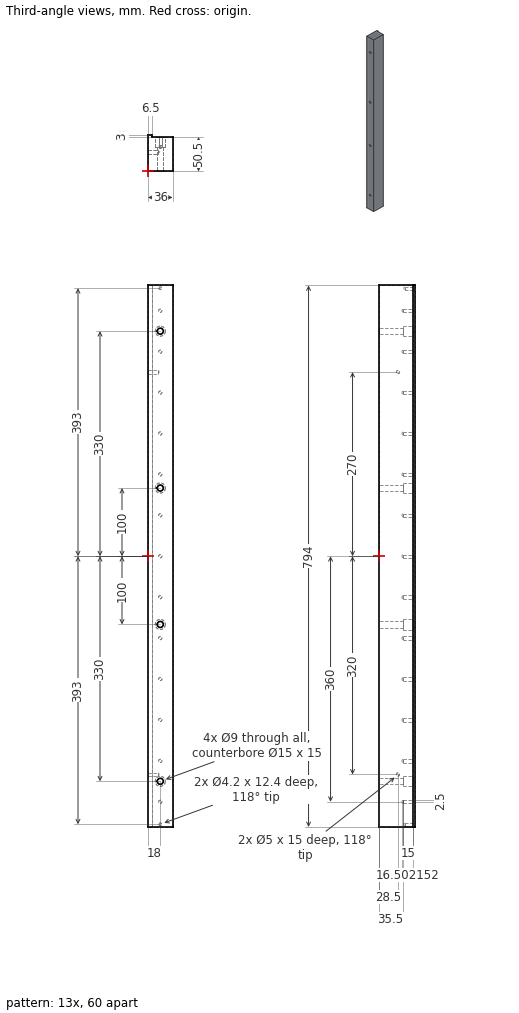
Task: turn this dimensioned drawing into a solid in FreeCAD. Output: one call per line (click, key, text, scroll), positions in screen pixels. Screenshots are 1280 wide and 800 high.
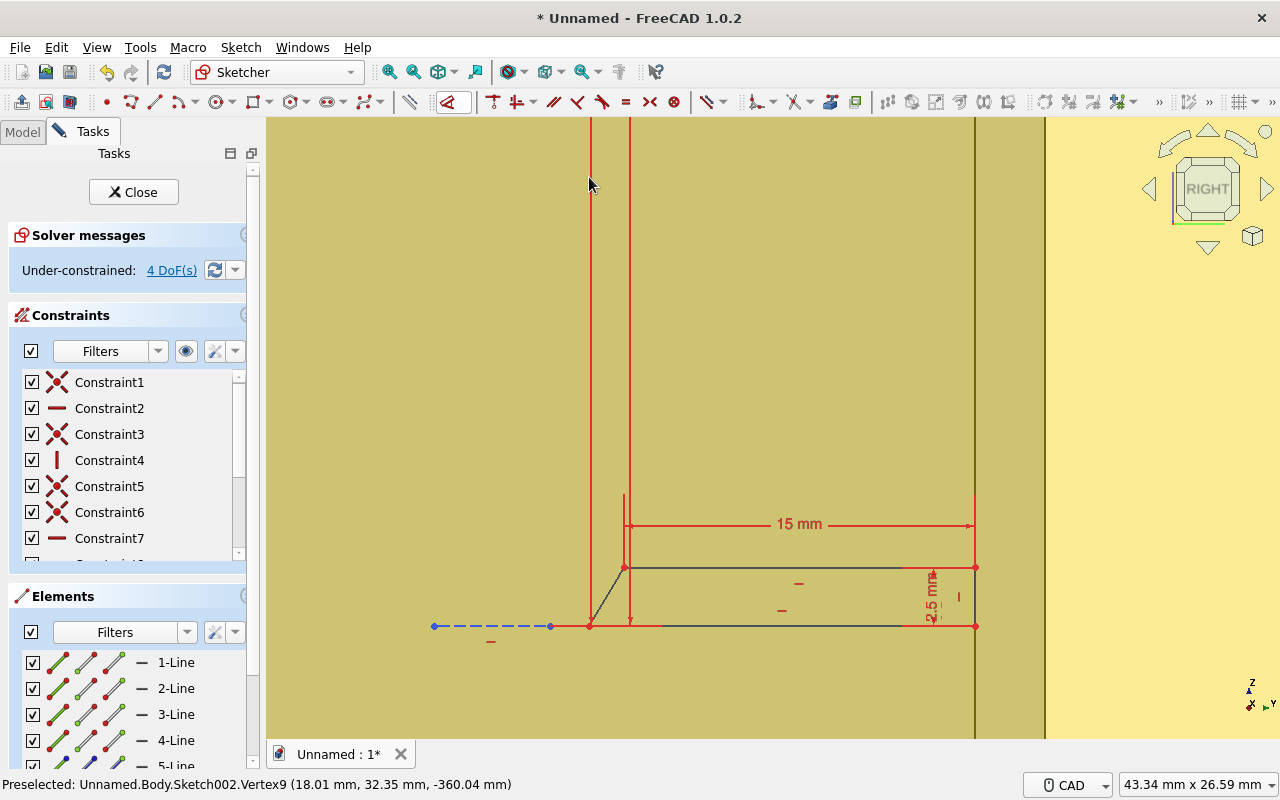
click(624, 568)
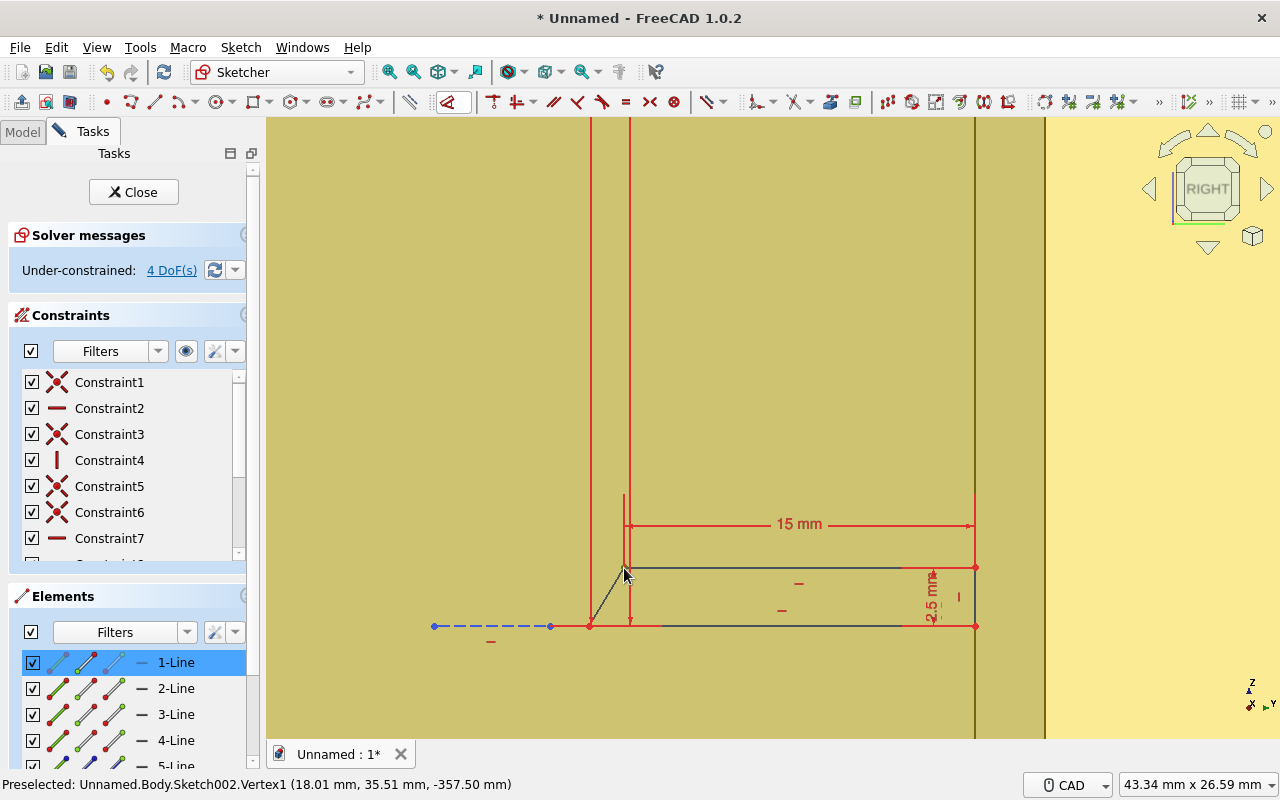
key(l)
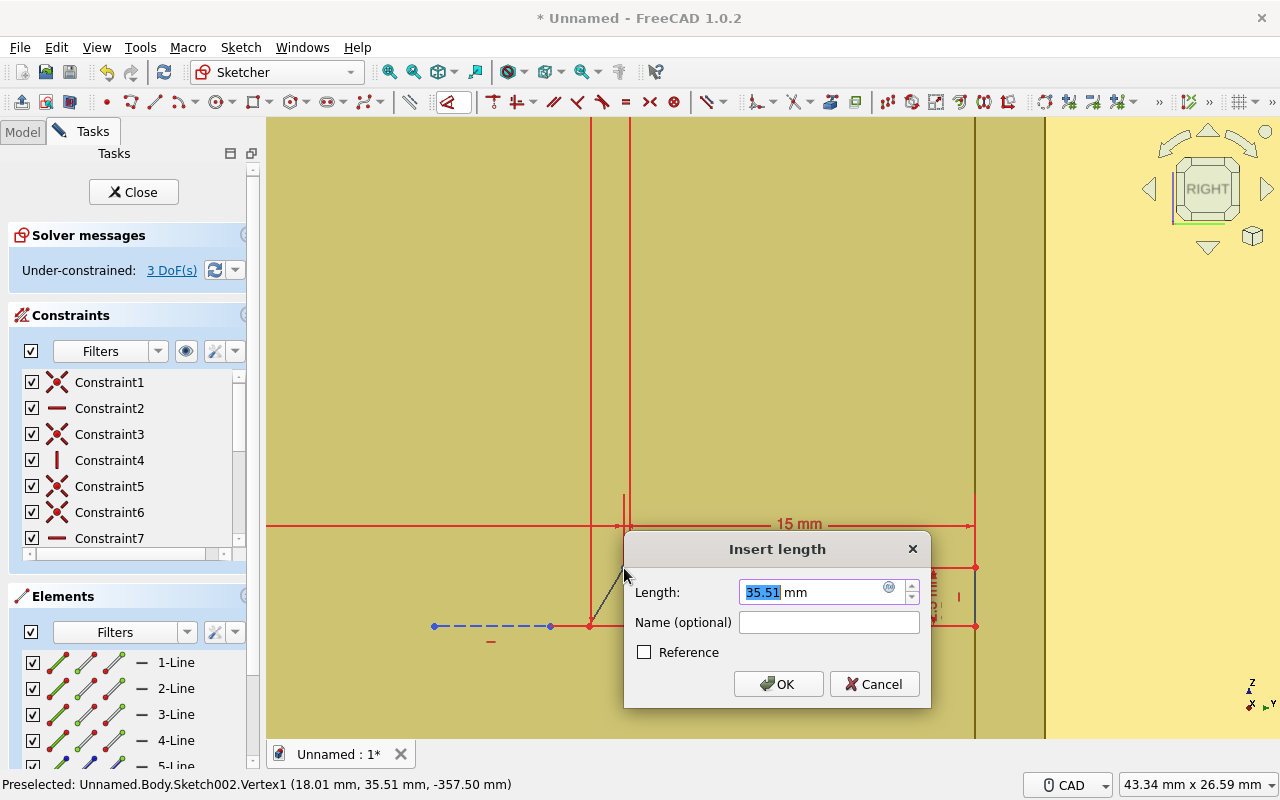
text(35.5)
key(Return)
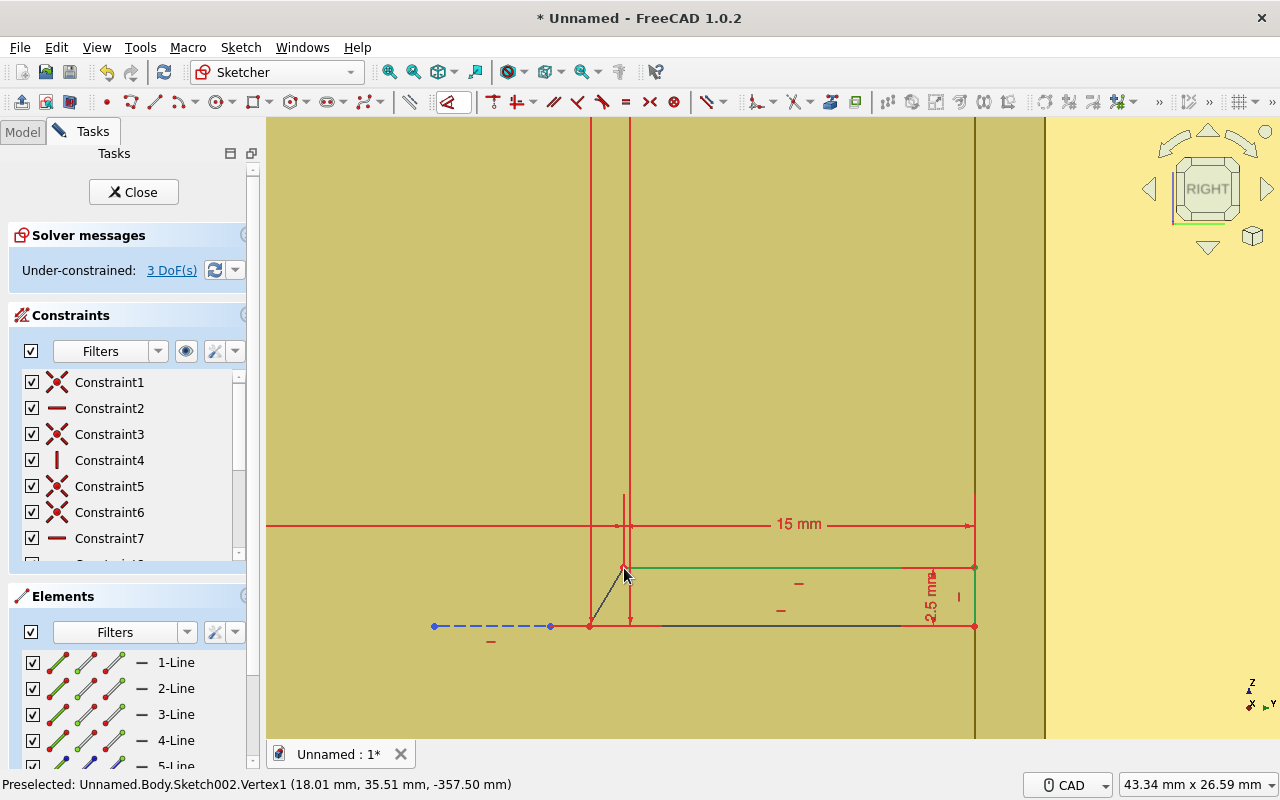
click(705, 626)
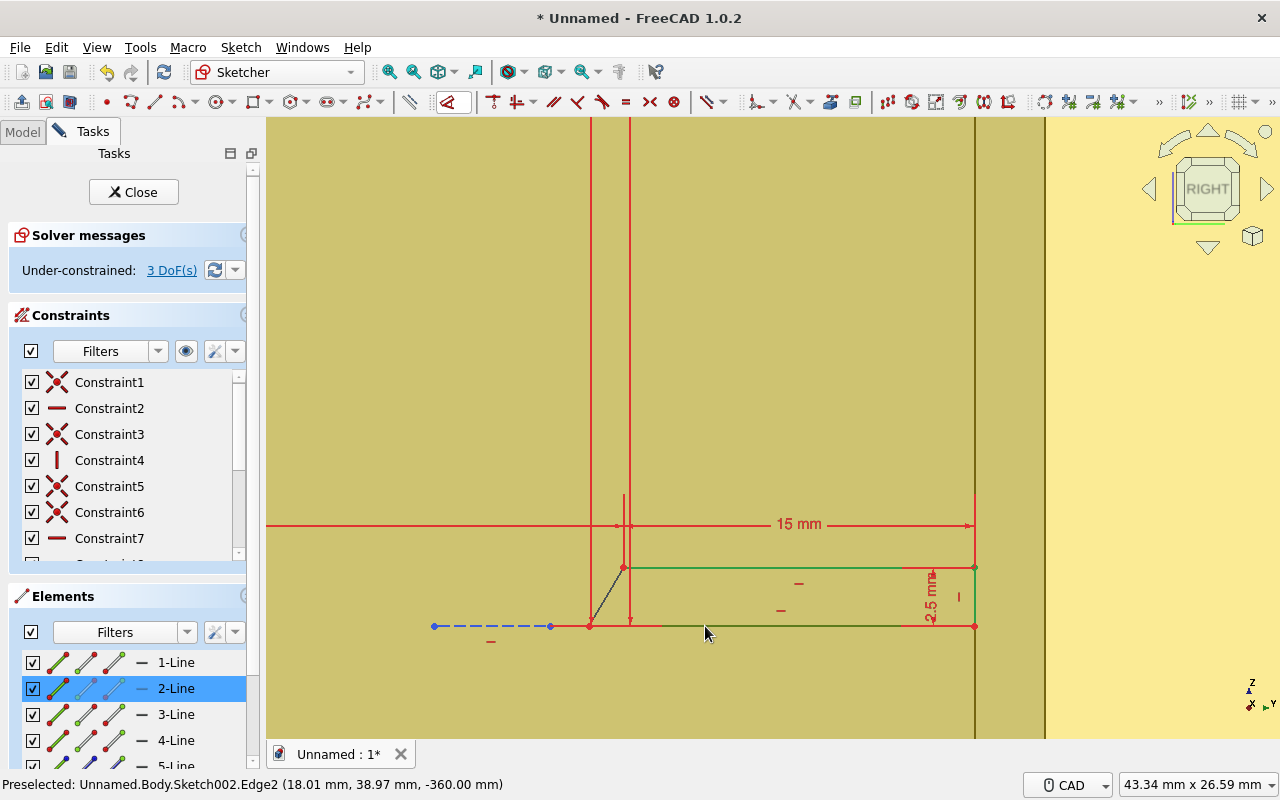
click(466, 102)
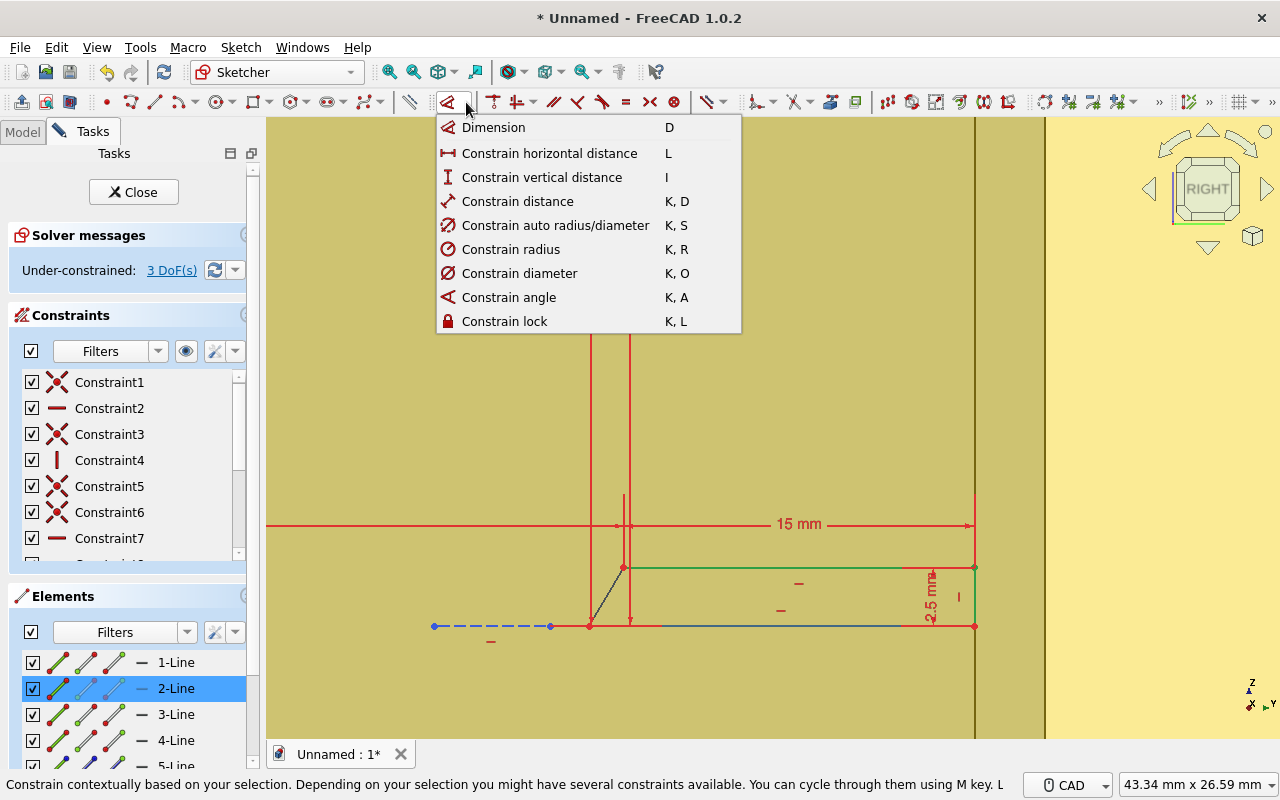
click(589, 153)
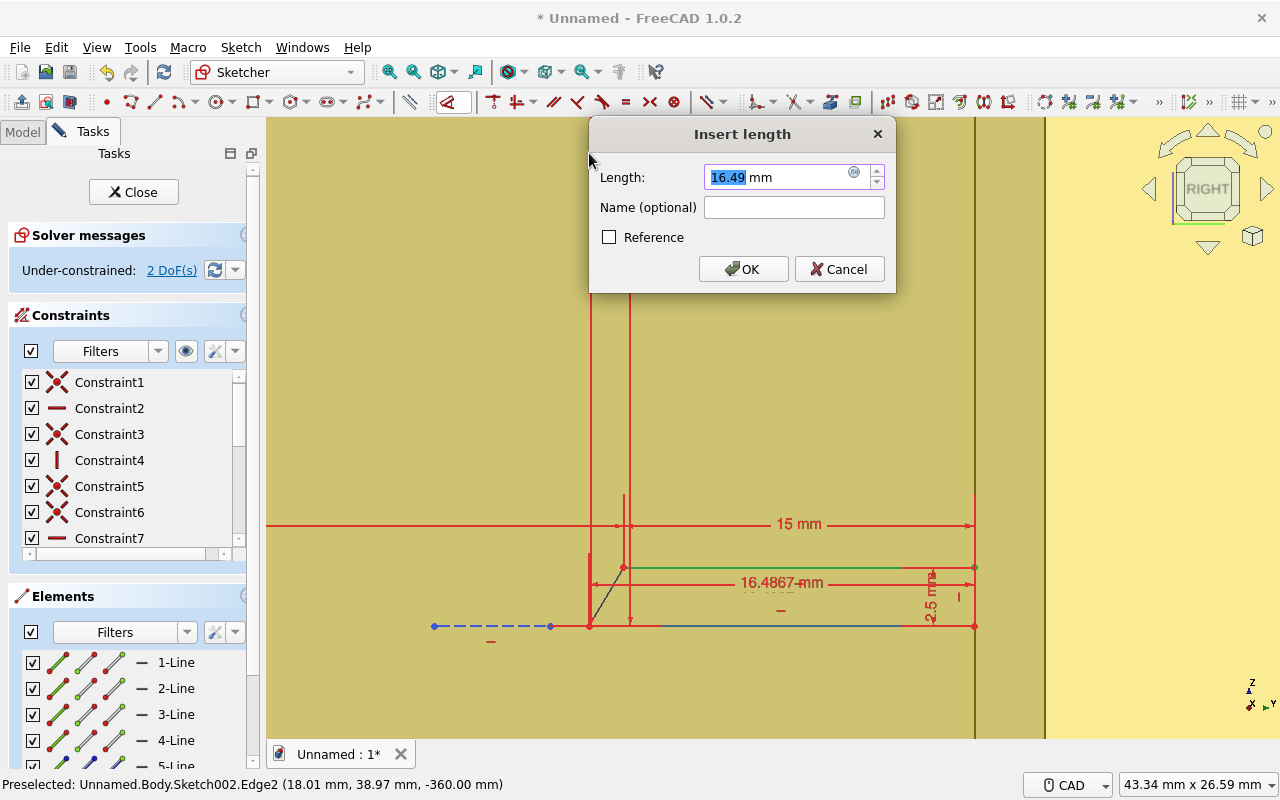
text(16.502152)
key(Return)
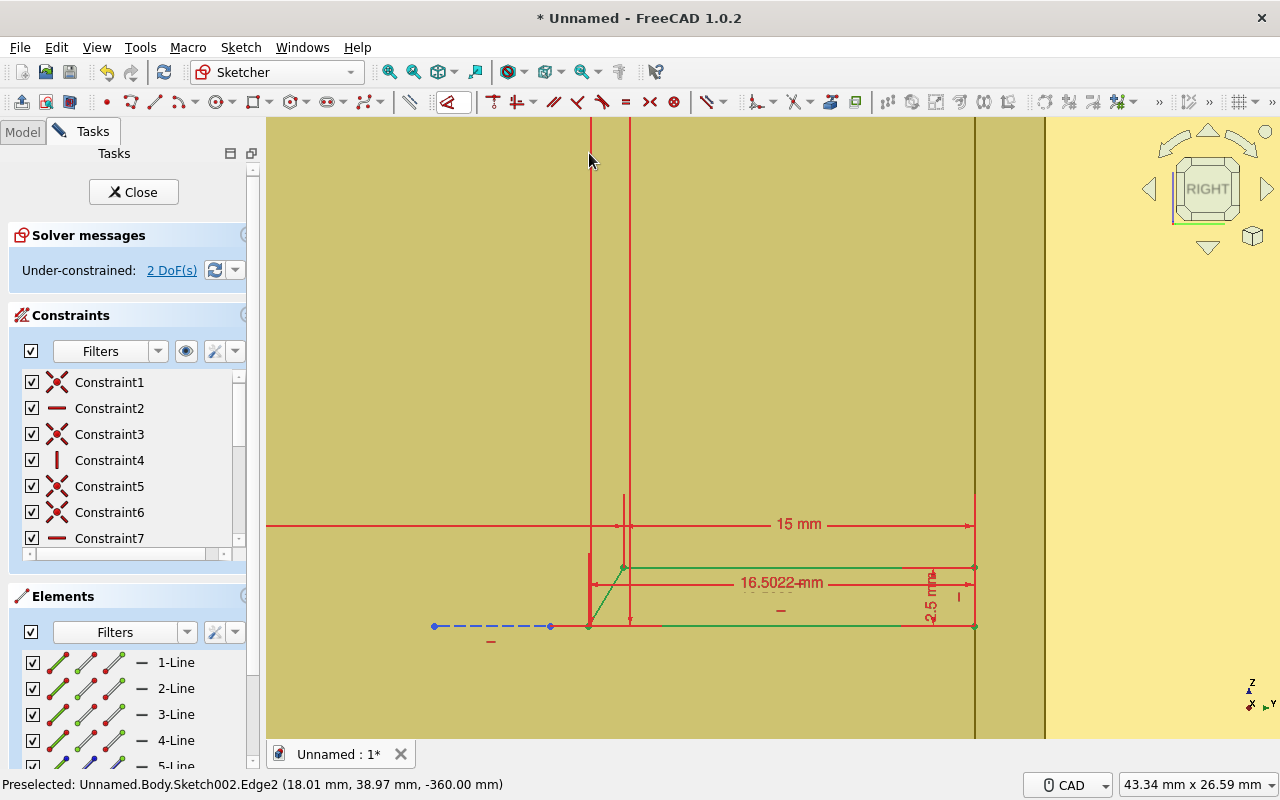
click(134, 192)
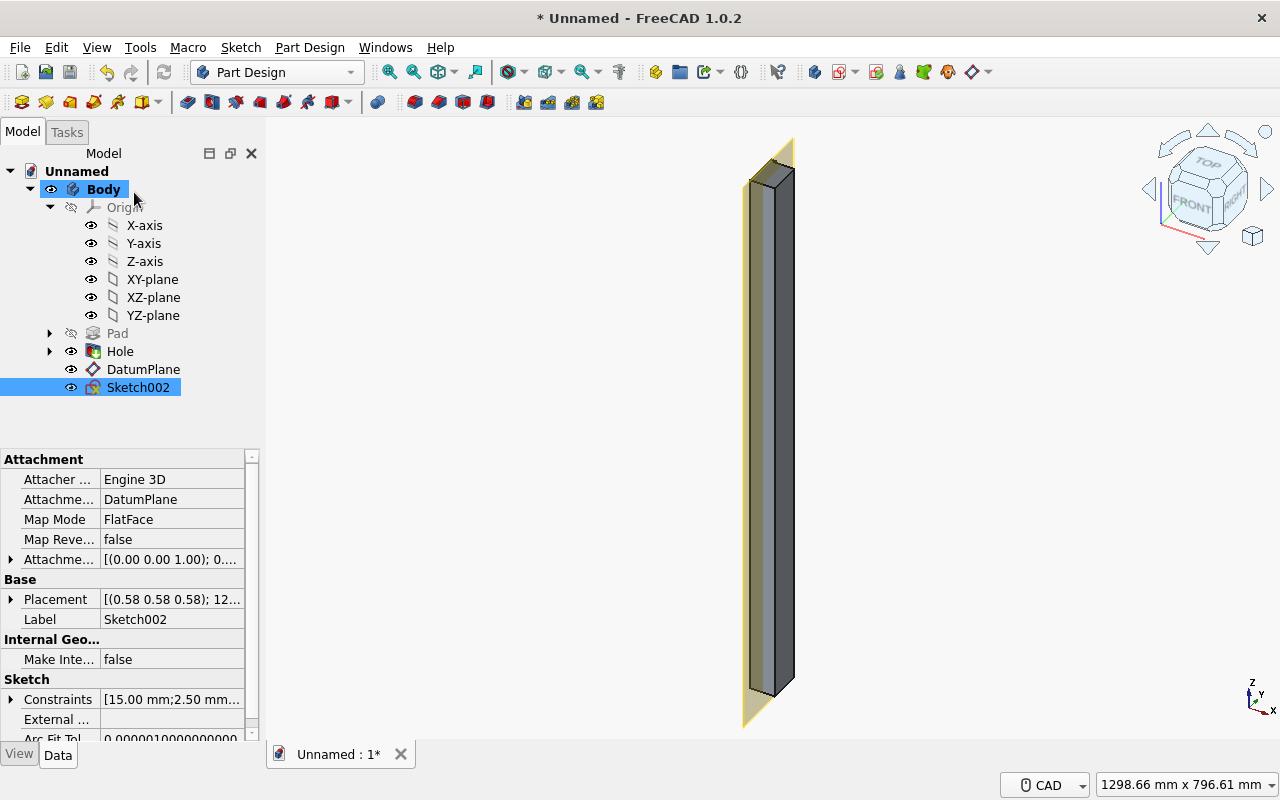
click(236, 102)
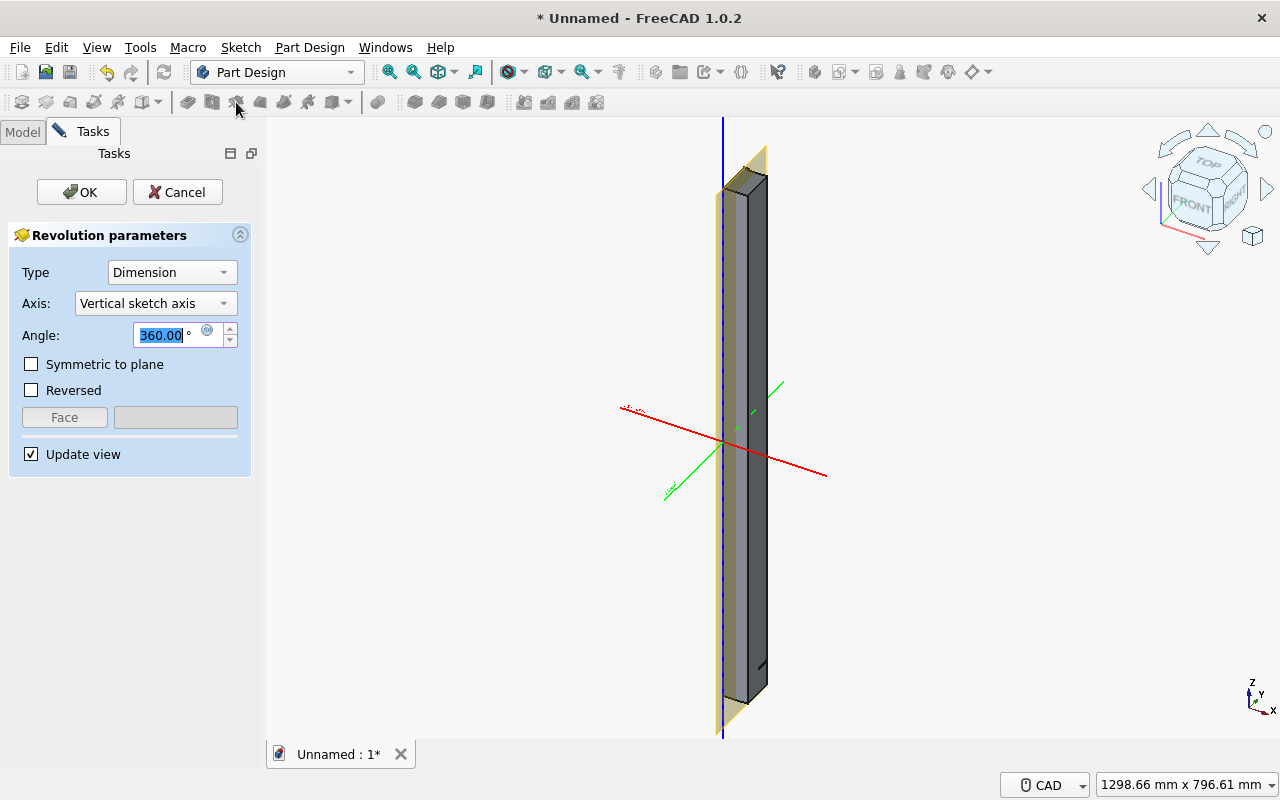
click(156, 304)